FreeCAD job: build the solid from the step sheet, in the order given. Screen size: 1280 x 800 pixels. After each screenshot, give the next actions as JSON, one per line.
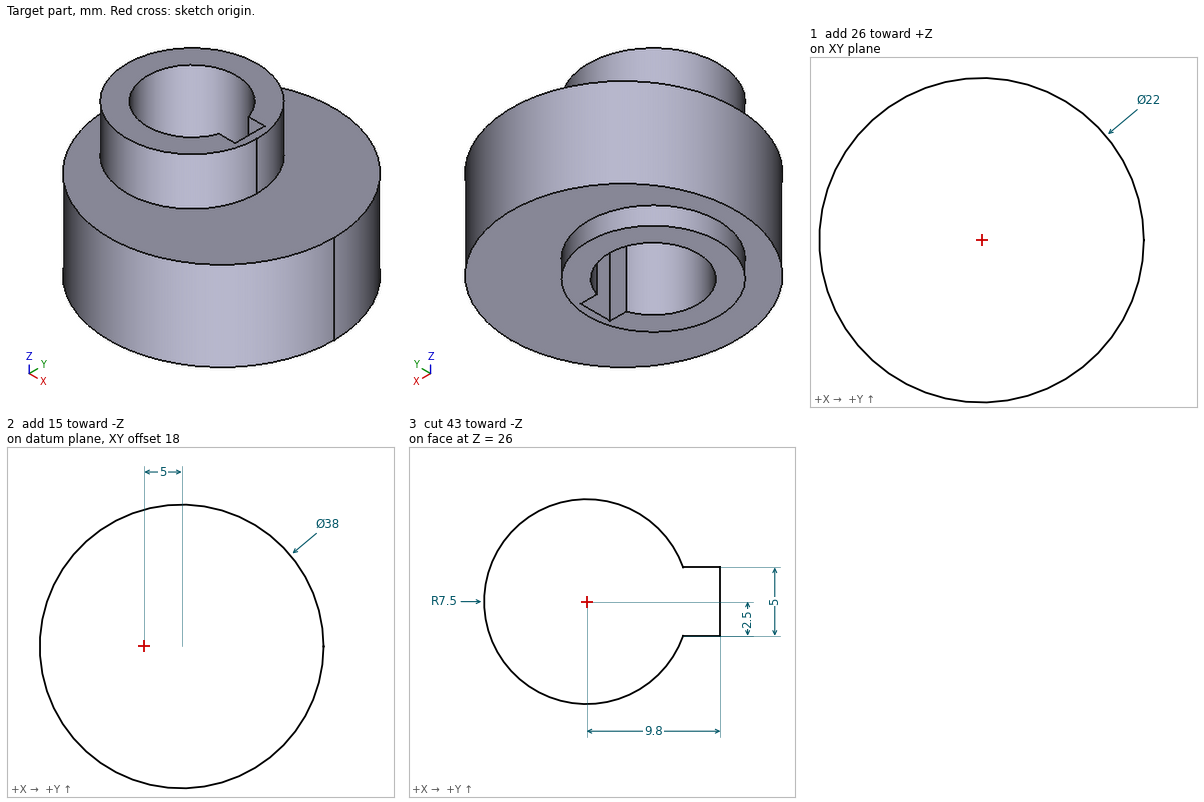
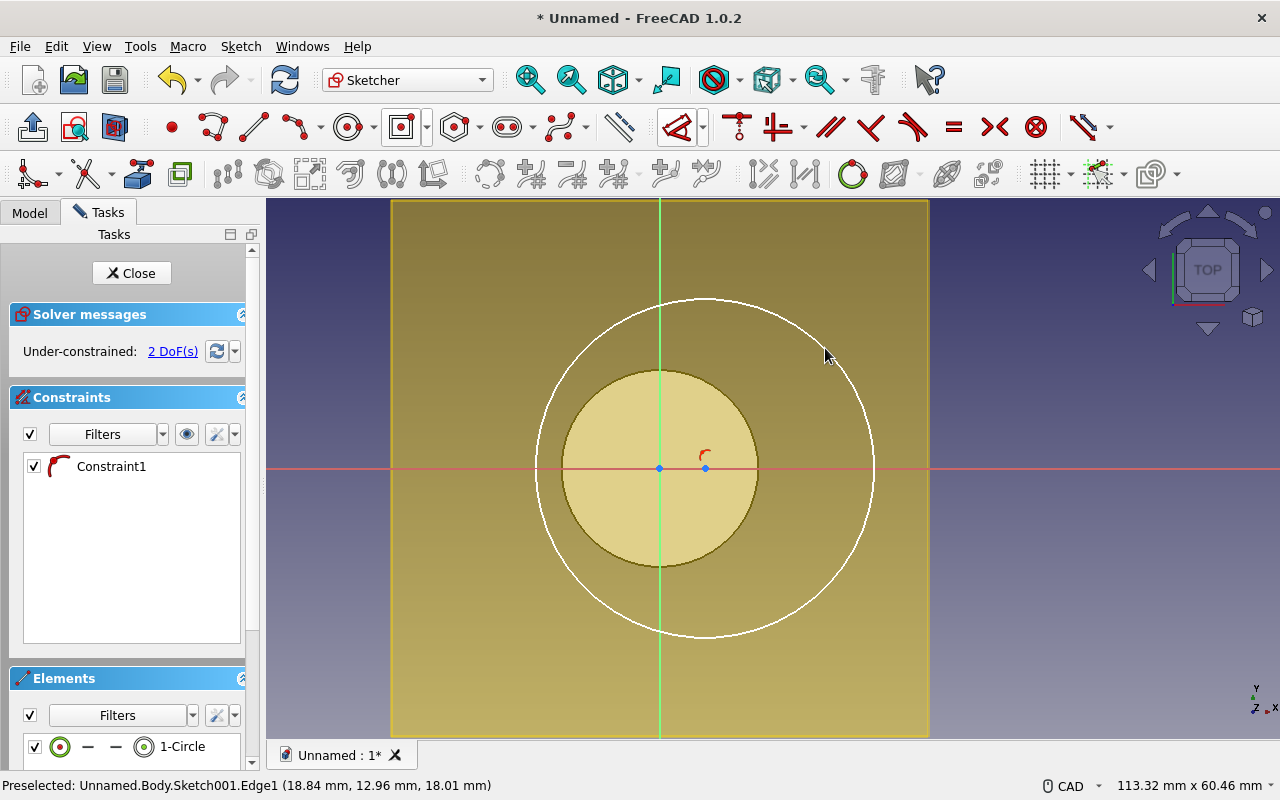
{"action": "key", "text": "d"}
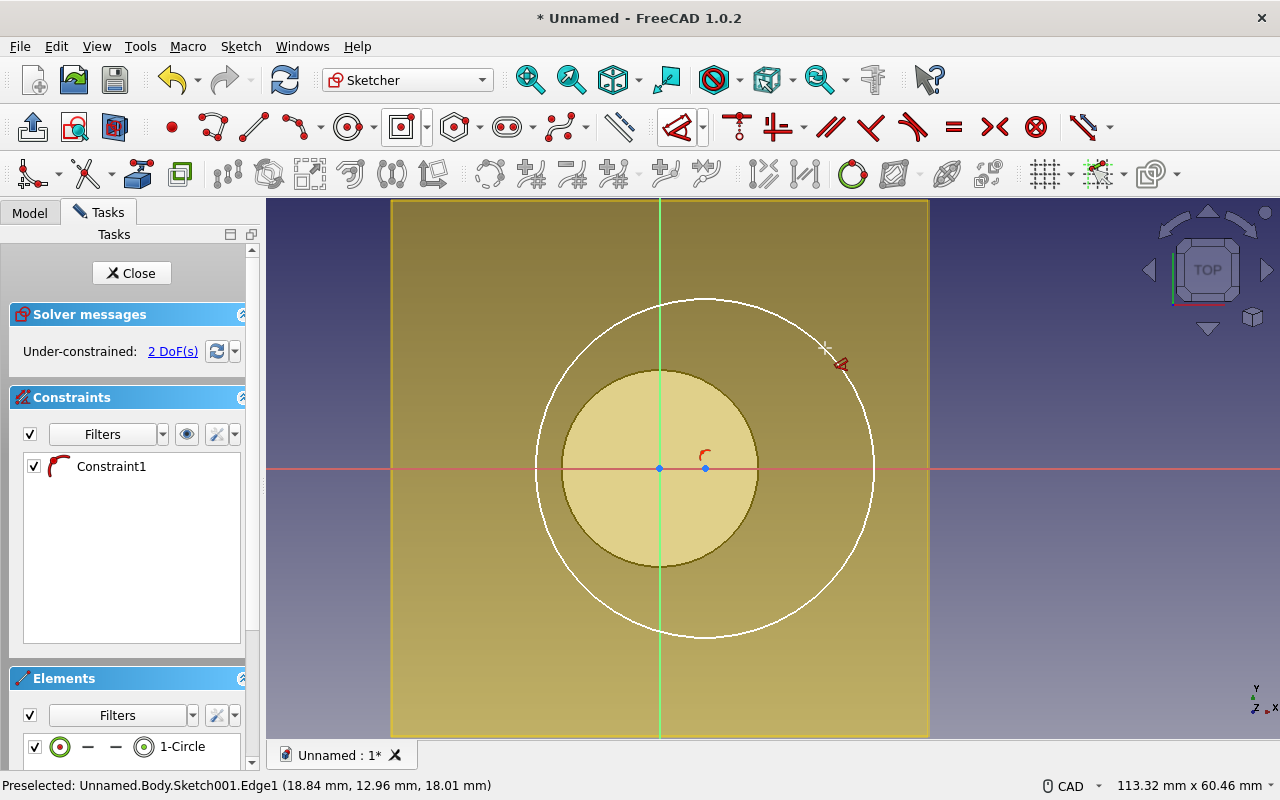
{"action": "left_click", "coordinate": [824, 348]}
{"action": "left_click", "coordinate": [846, 325]}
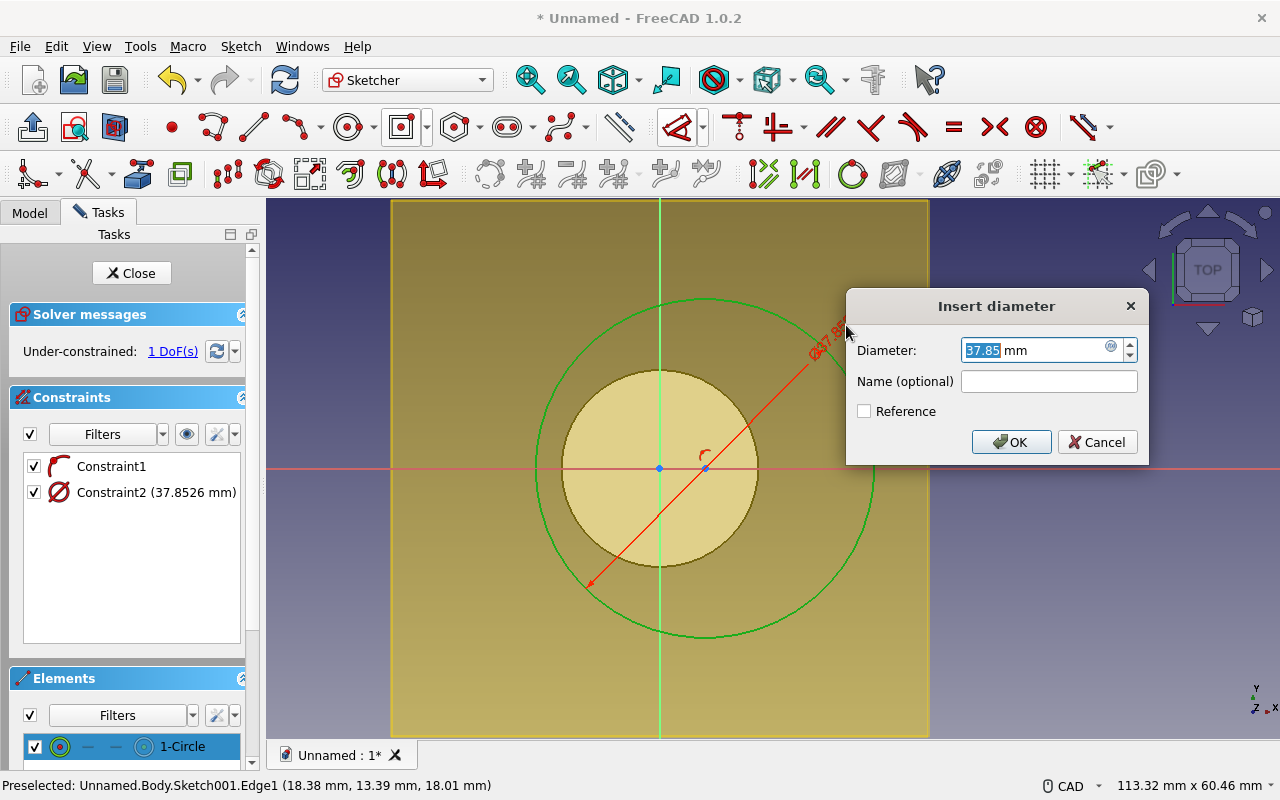
{"action": "type", "text": "38"}
{"action": "key", "text": "Return"}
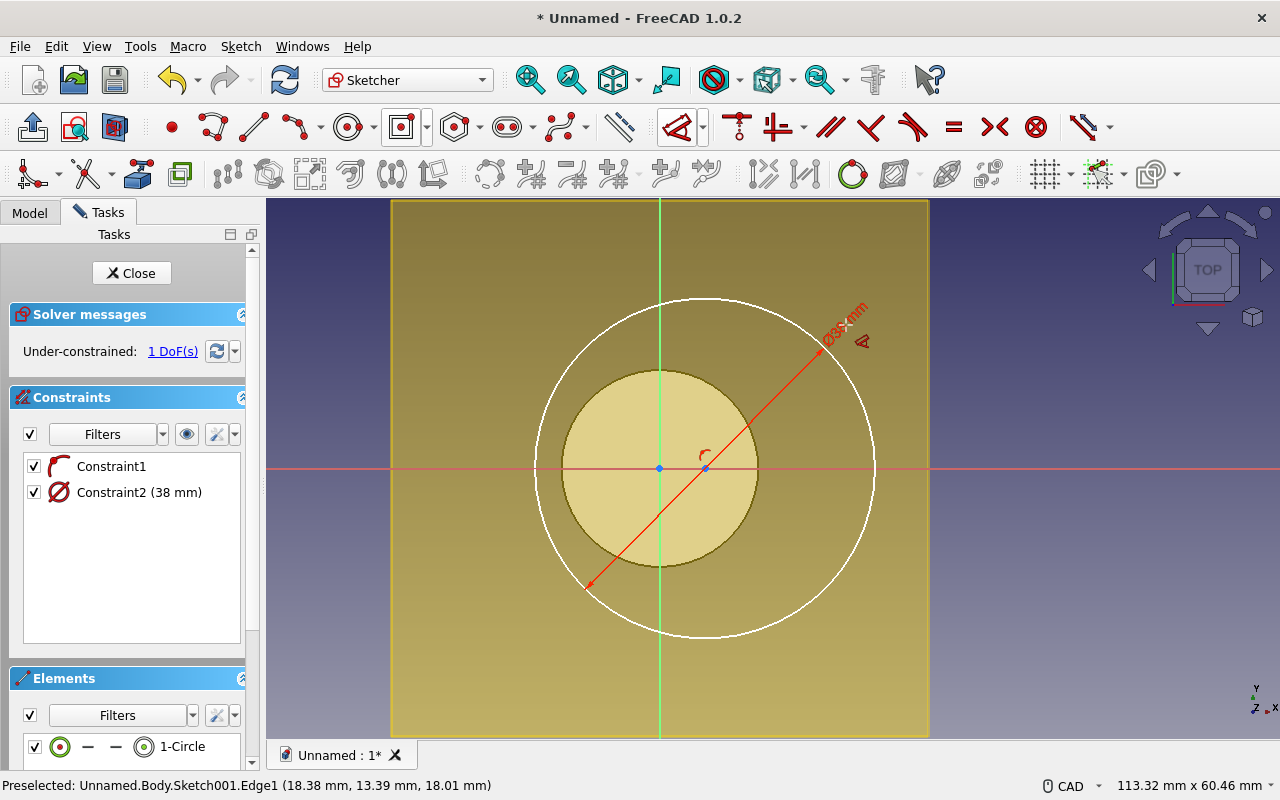
{"action": "left_click", "coordinate": [705, 468]}
{"action": "left_click", "coordinate": [682, 502]}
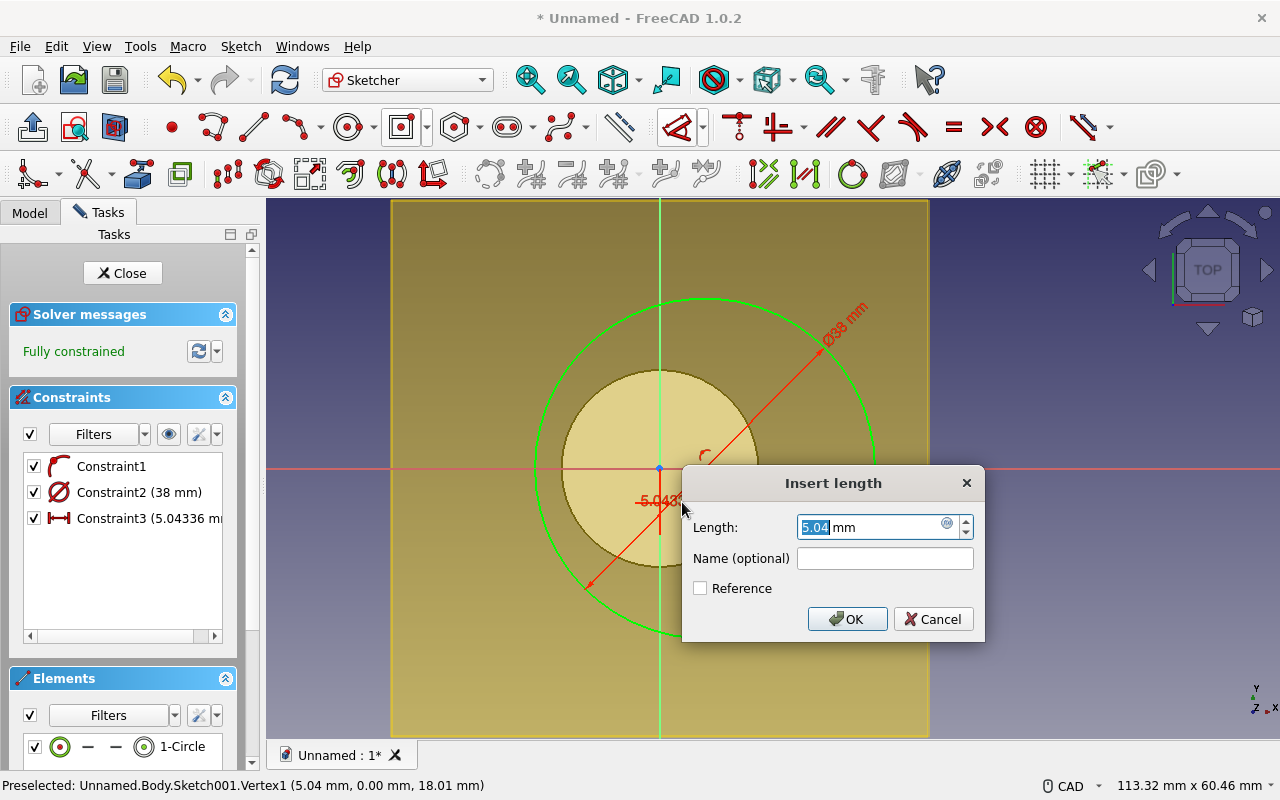
{"action": "type", "text": "5"}
{"action": "key", "text": "Return"}
{"action": "key", "text": "Escape"}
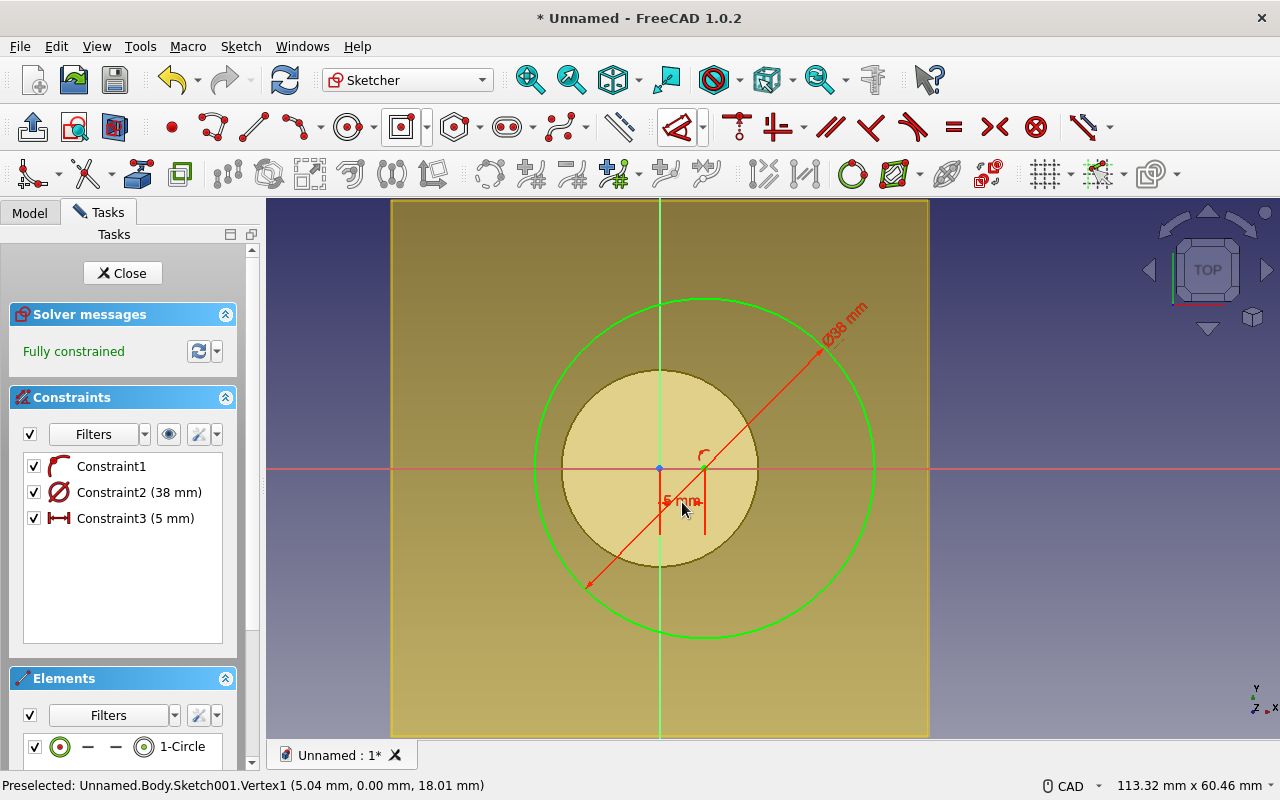
{"action": "left_click", "coordinate": [123, 273]}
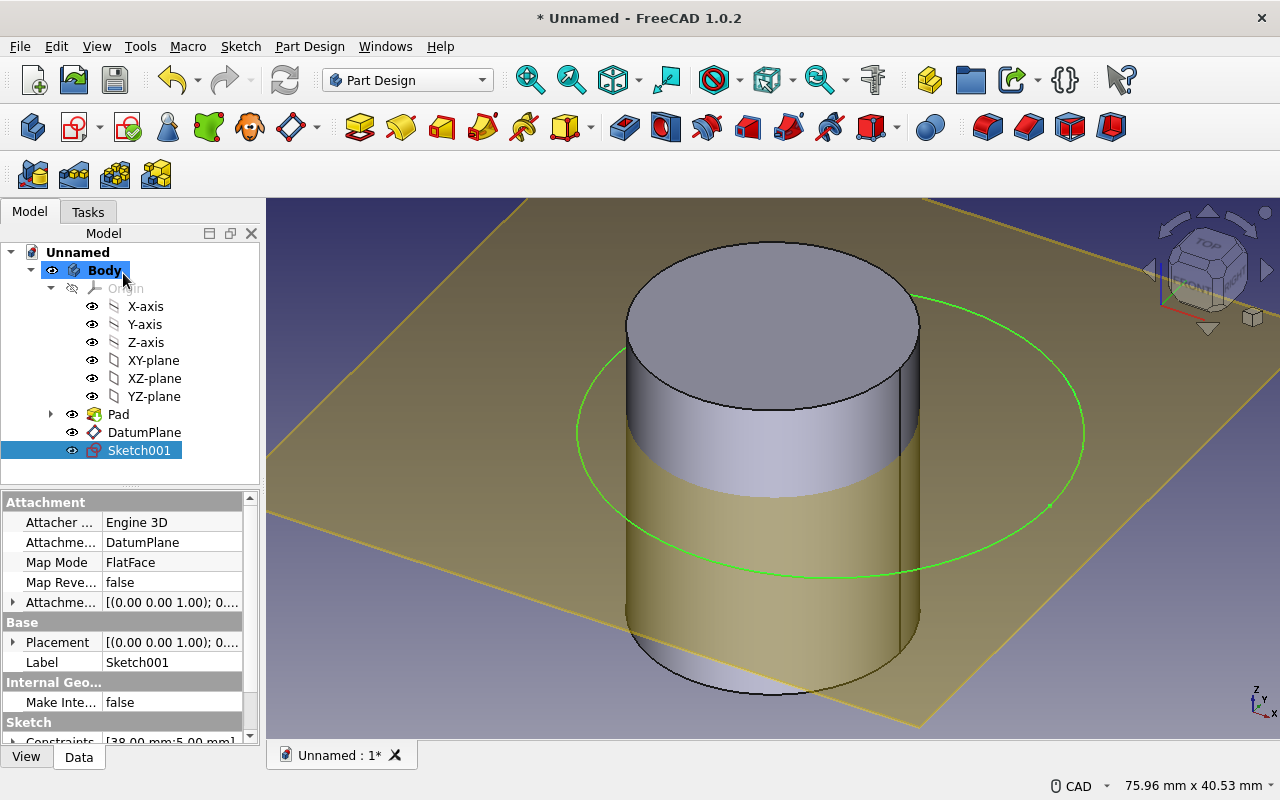
{"action": "left_click", "coordinate": [360, 128]}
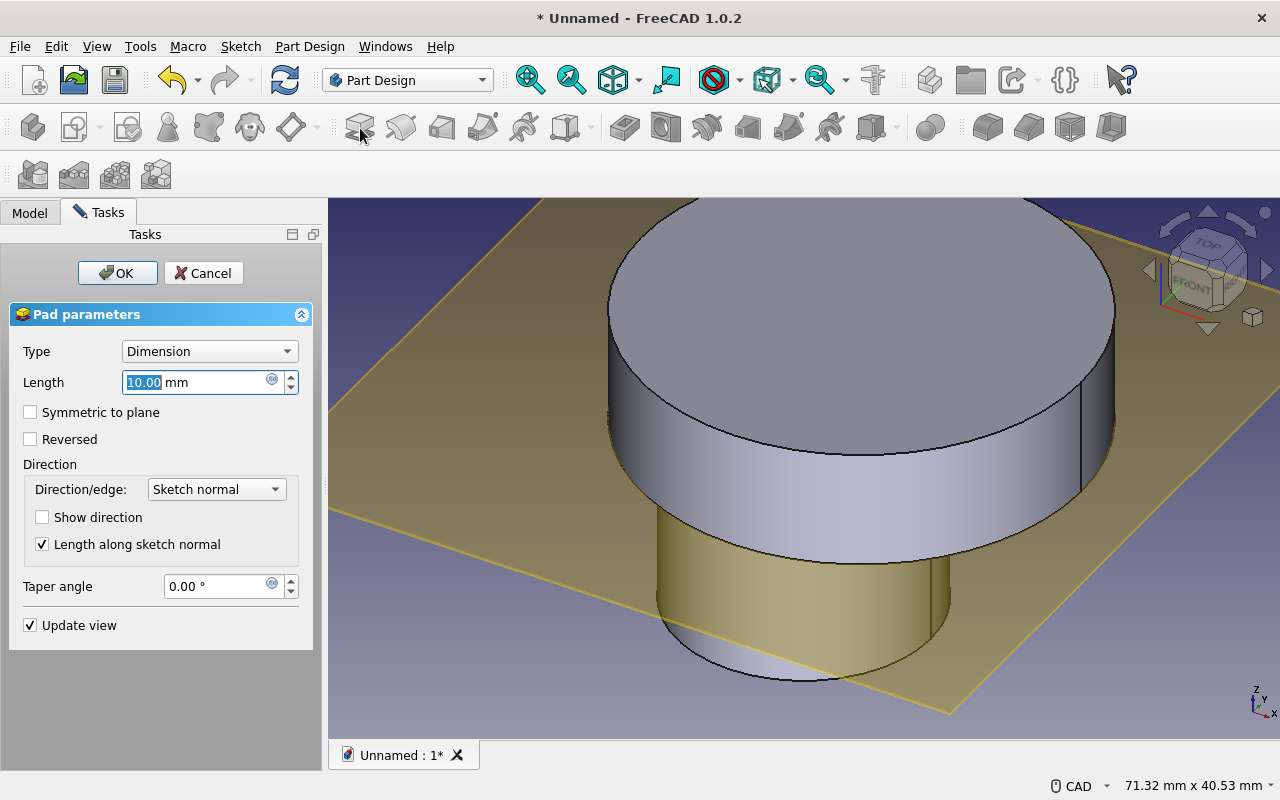
{"action": "type", "text": "15"}
{"action": "key", "text": "Tab"}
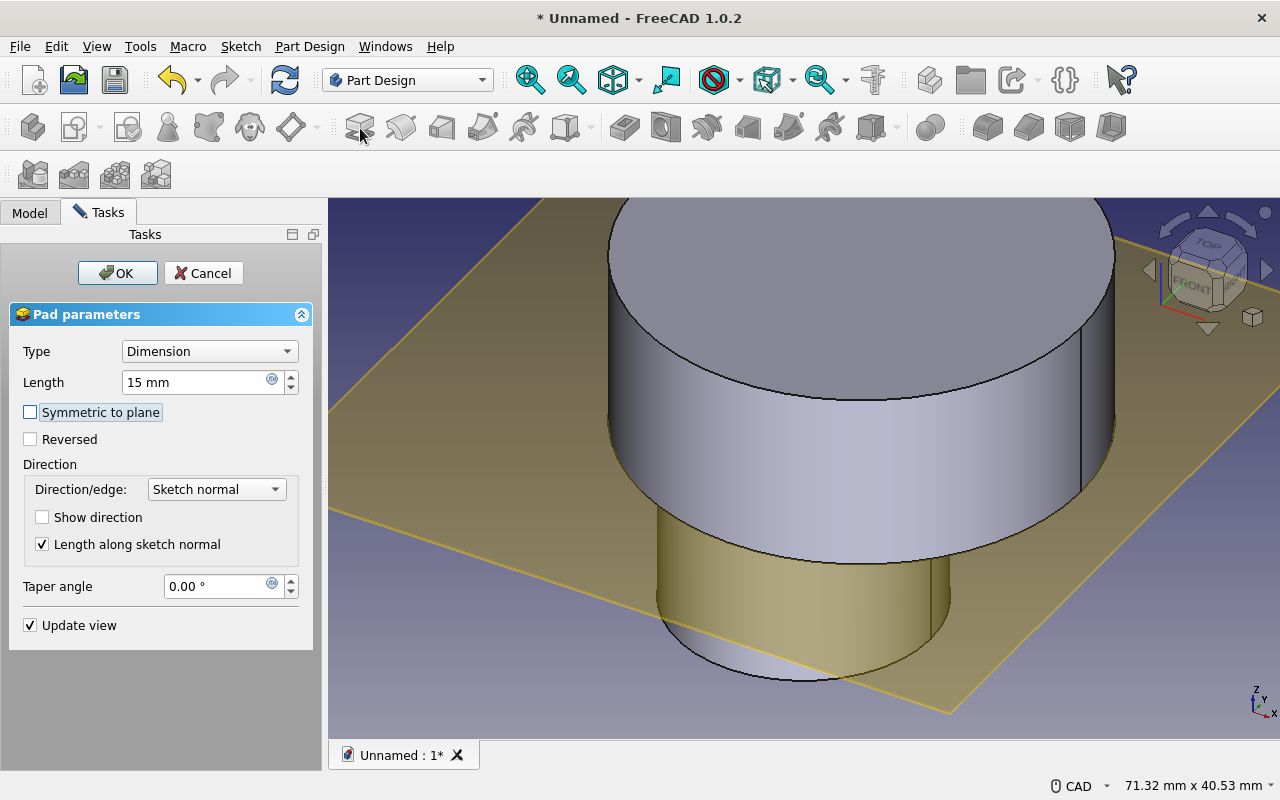
{"action": "left_click", "coordinate": [31, 439]}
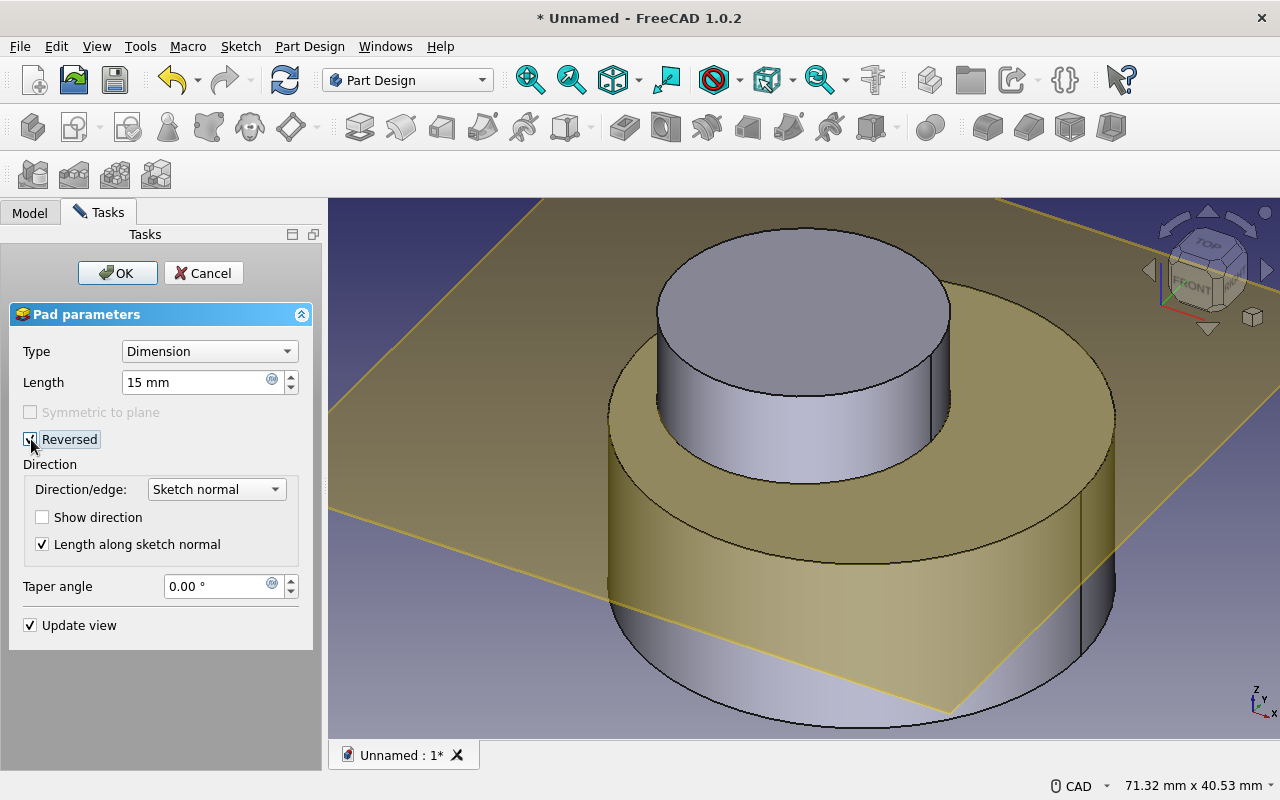
{"action": "left_click", "coordinate": [118, 273]}